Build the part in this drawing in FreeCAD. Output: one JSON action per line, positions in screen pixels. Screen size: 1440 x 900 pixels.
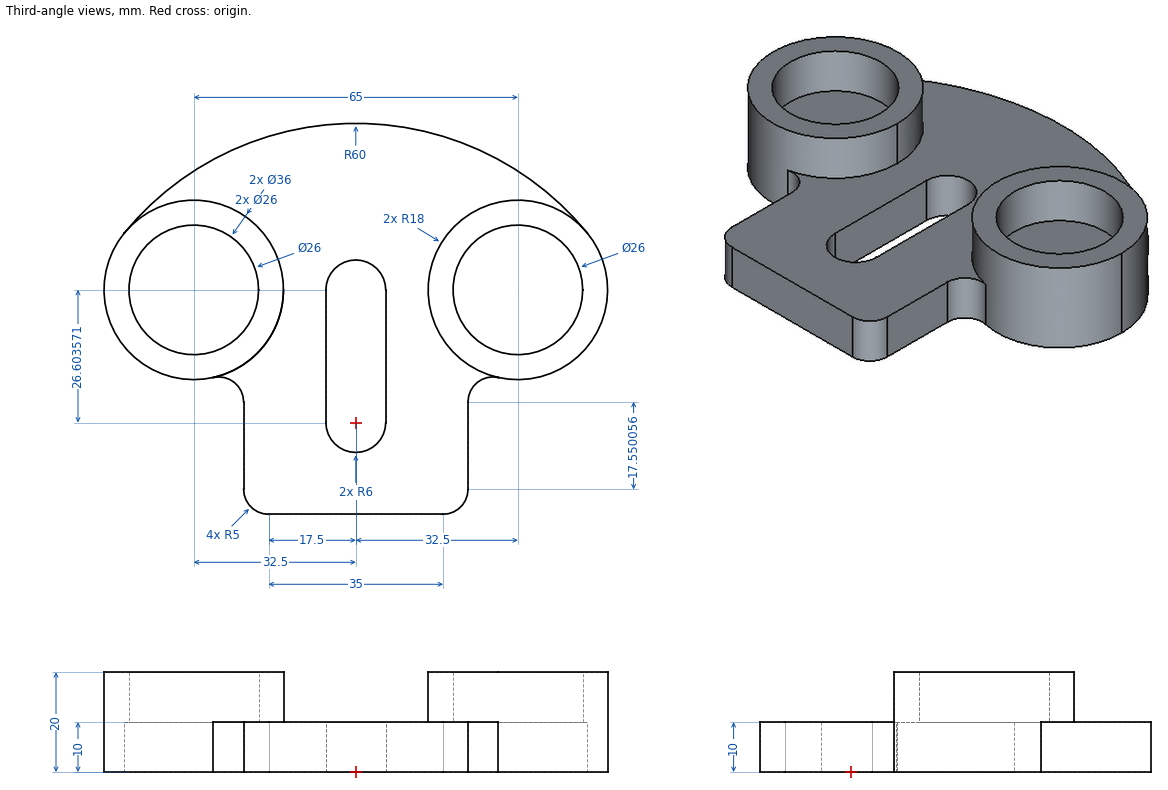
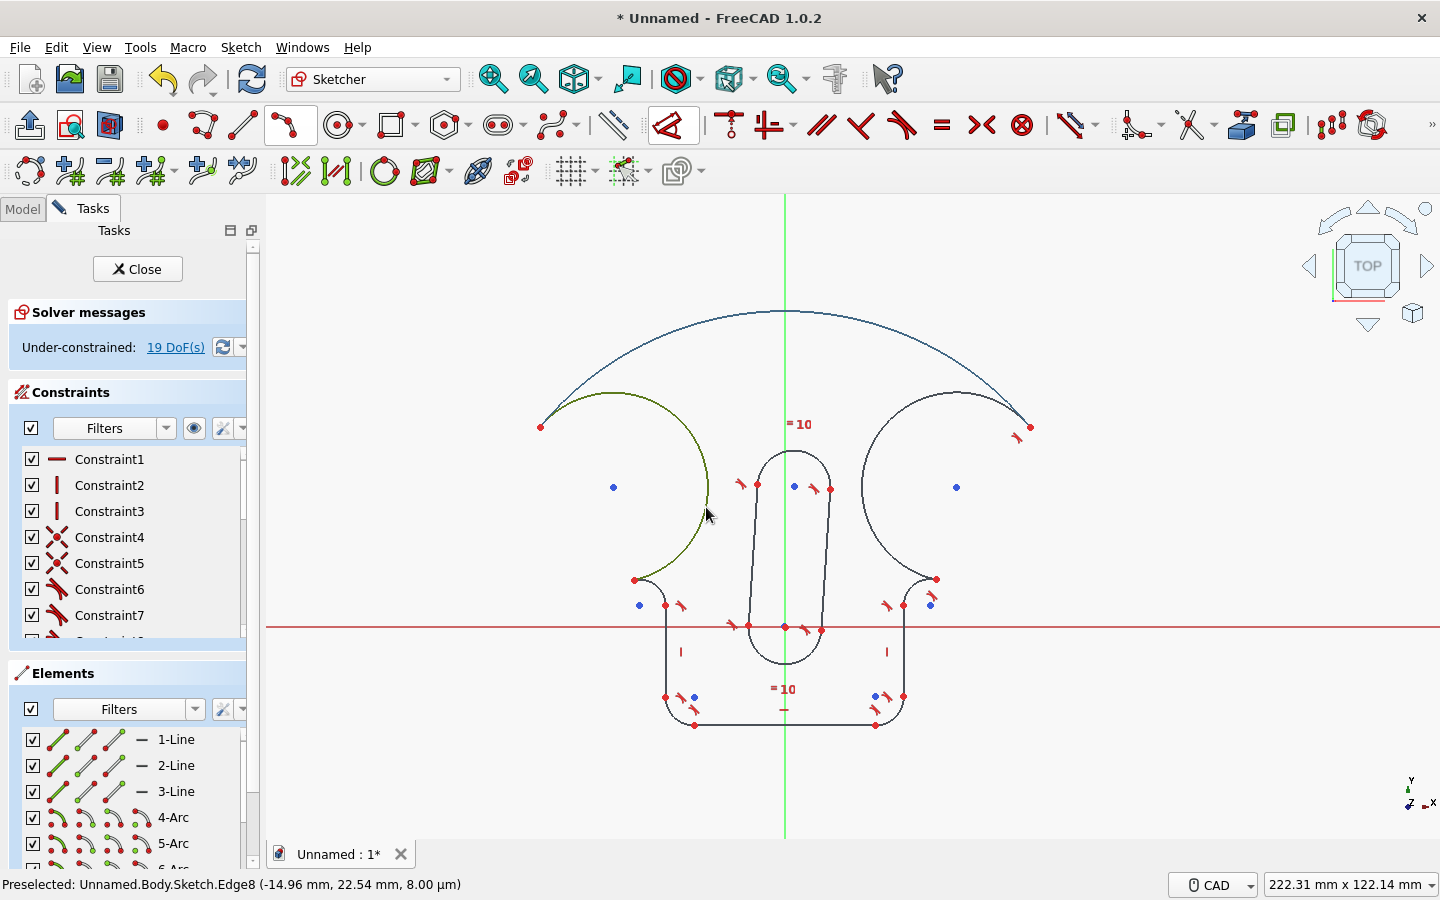
{"action": "left_click", "coordinate": [902, 126]}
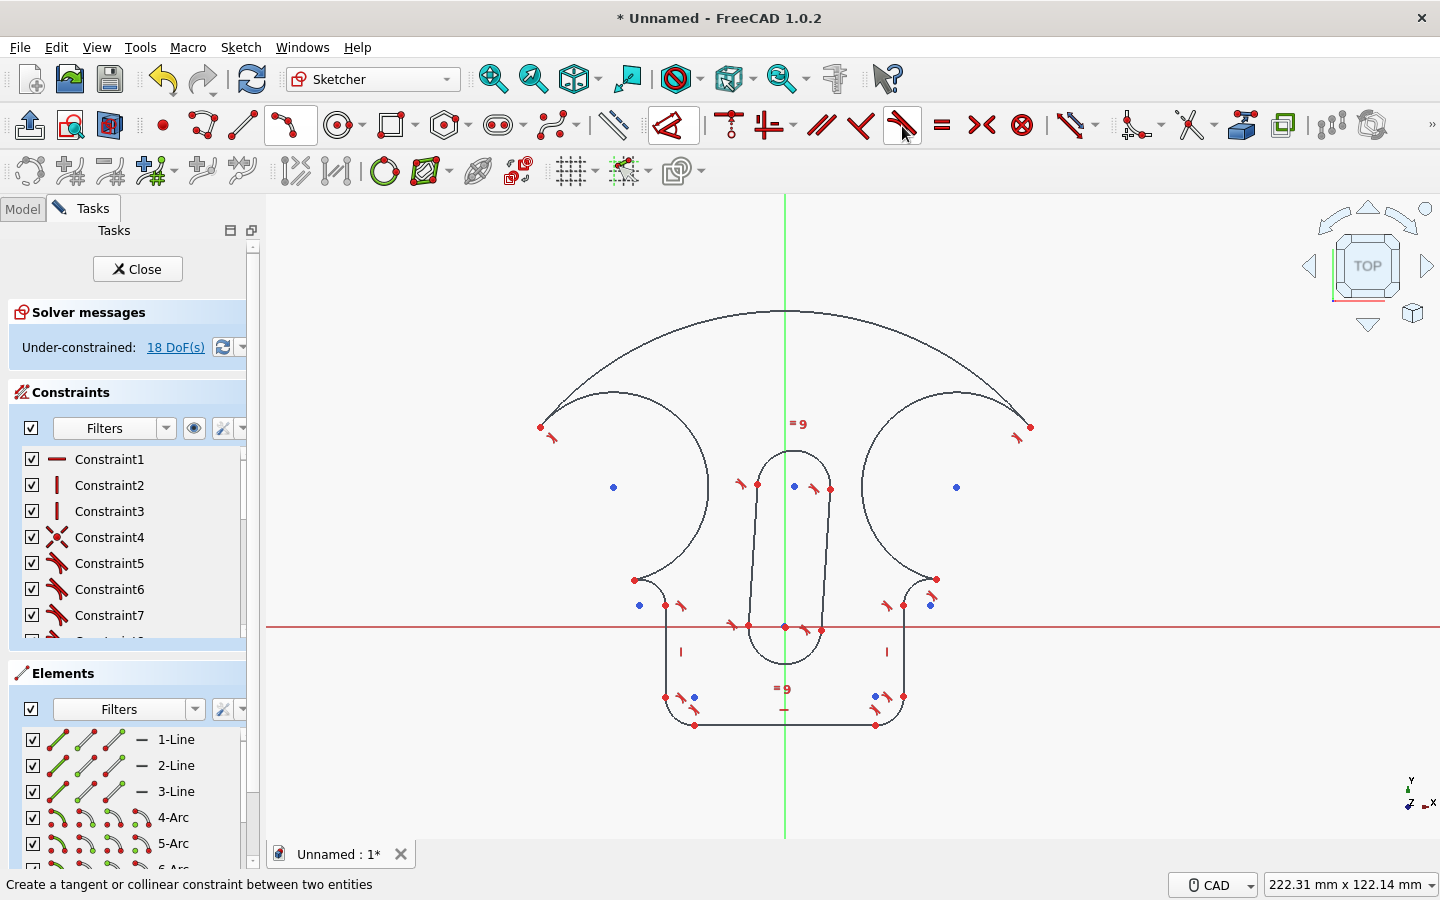
{"action": "left_click", "coordinate": [706, 507]}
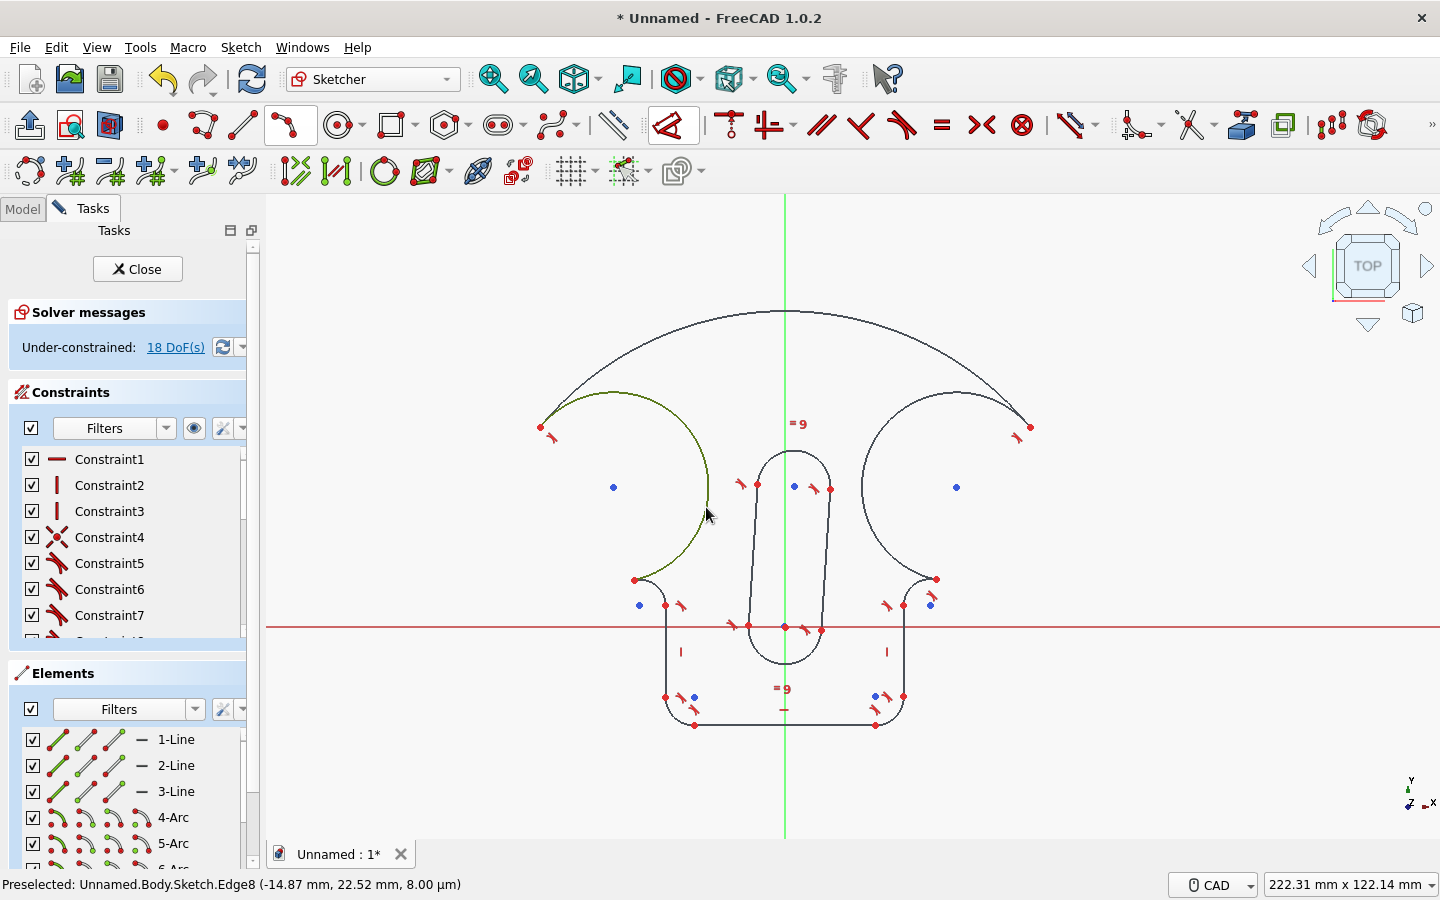
{"action": "left_click", "coordinate": [662, 592]}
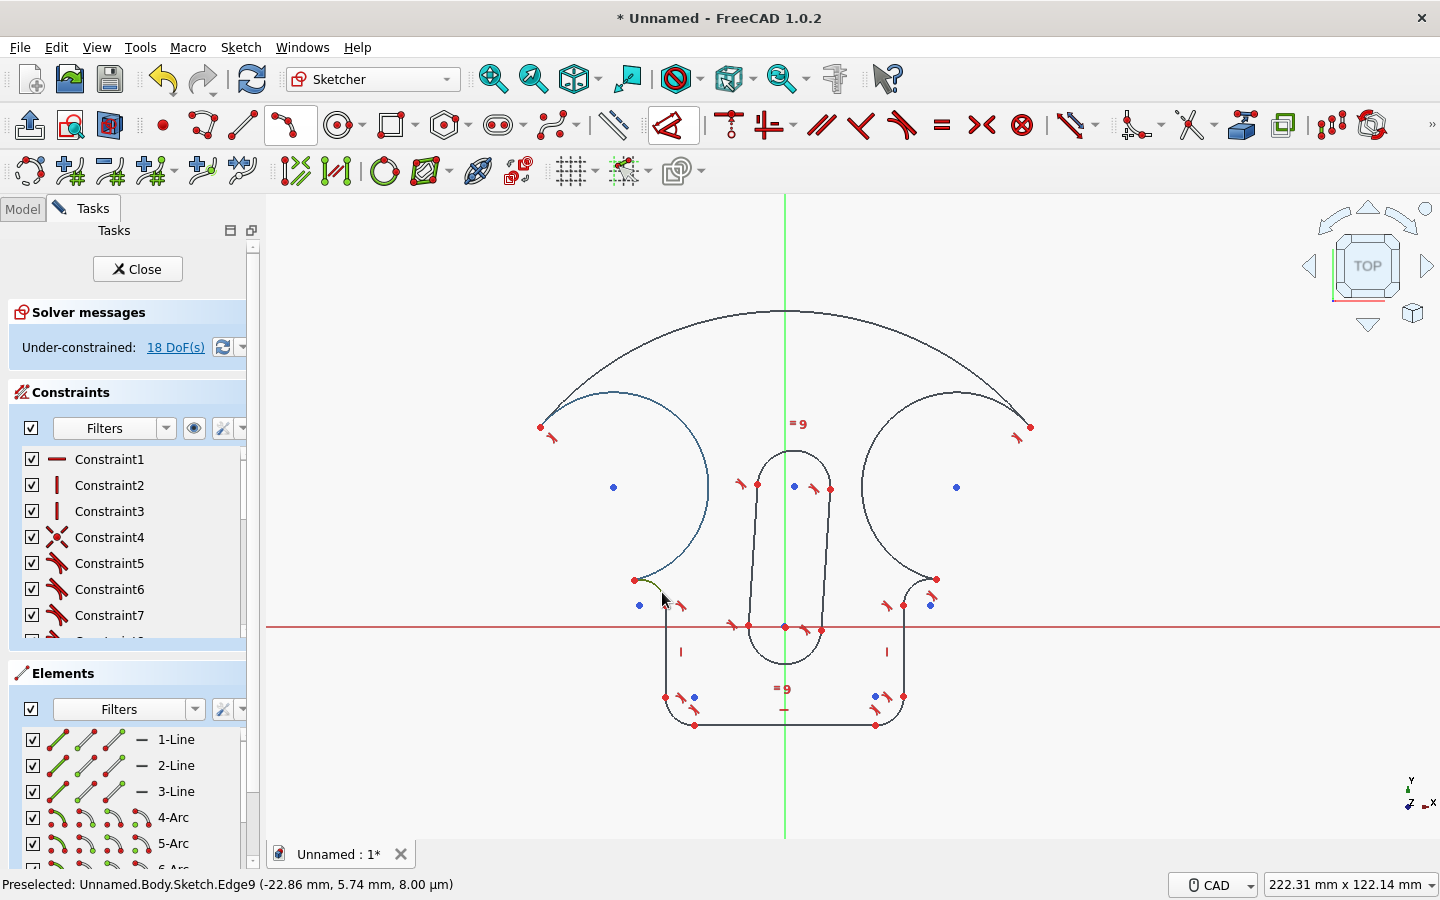
{"action": "left_click", "coordinate": [902, 126]}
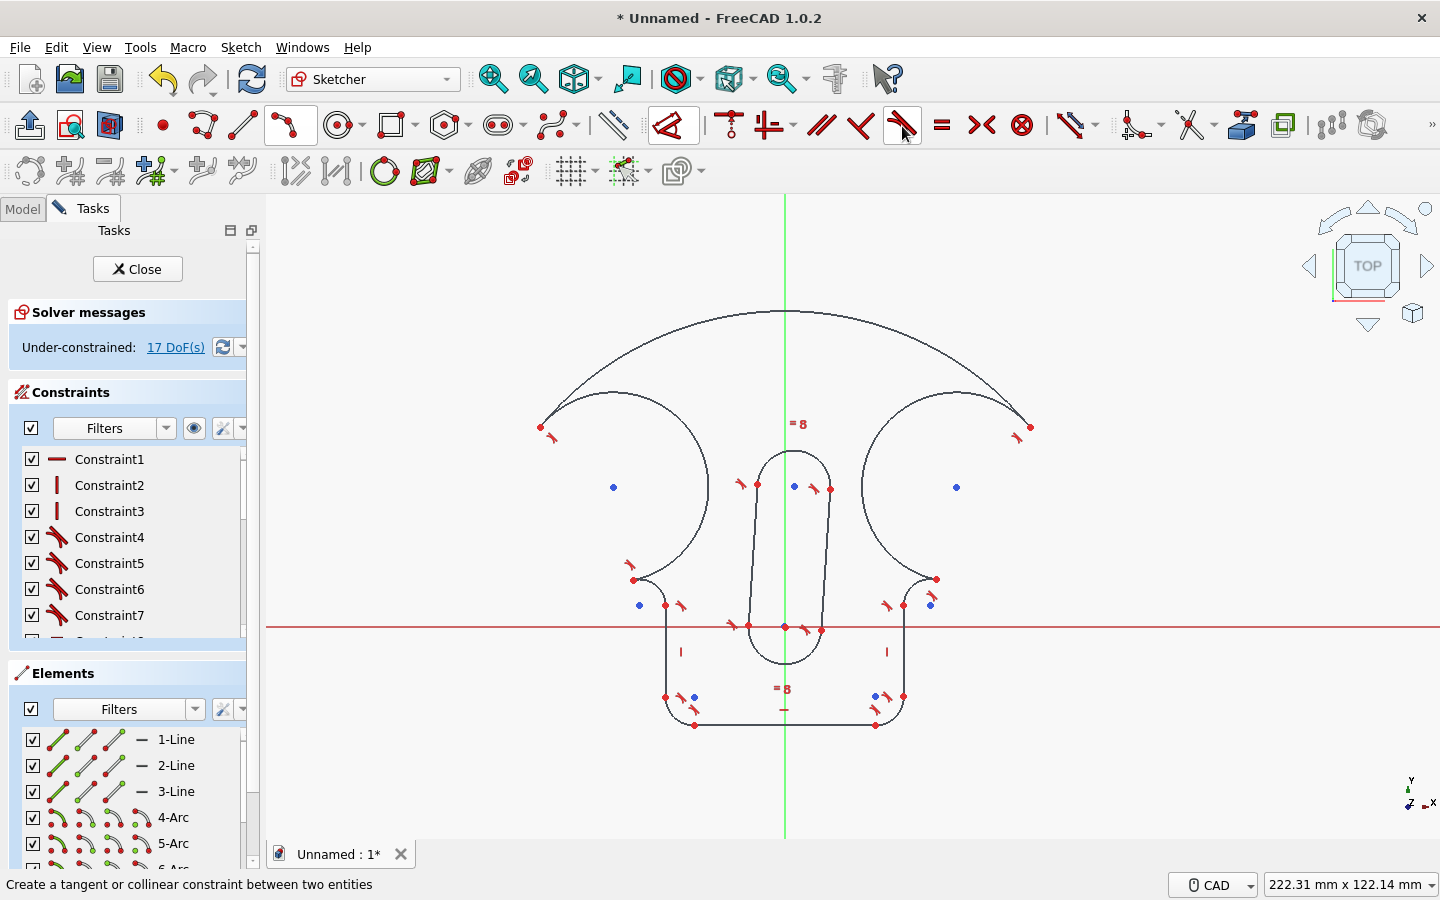
{"action": "left_click", "coordinate": [751, 583]}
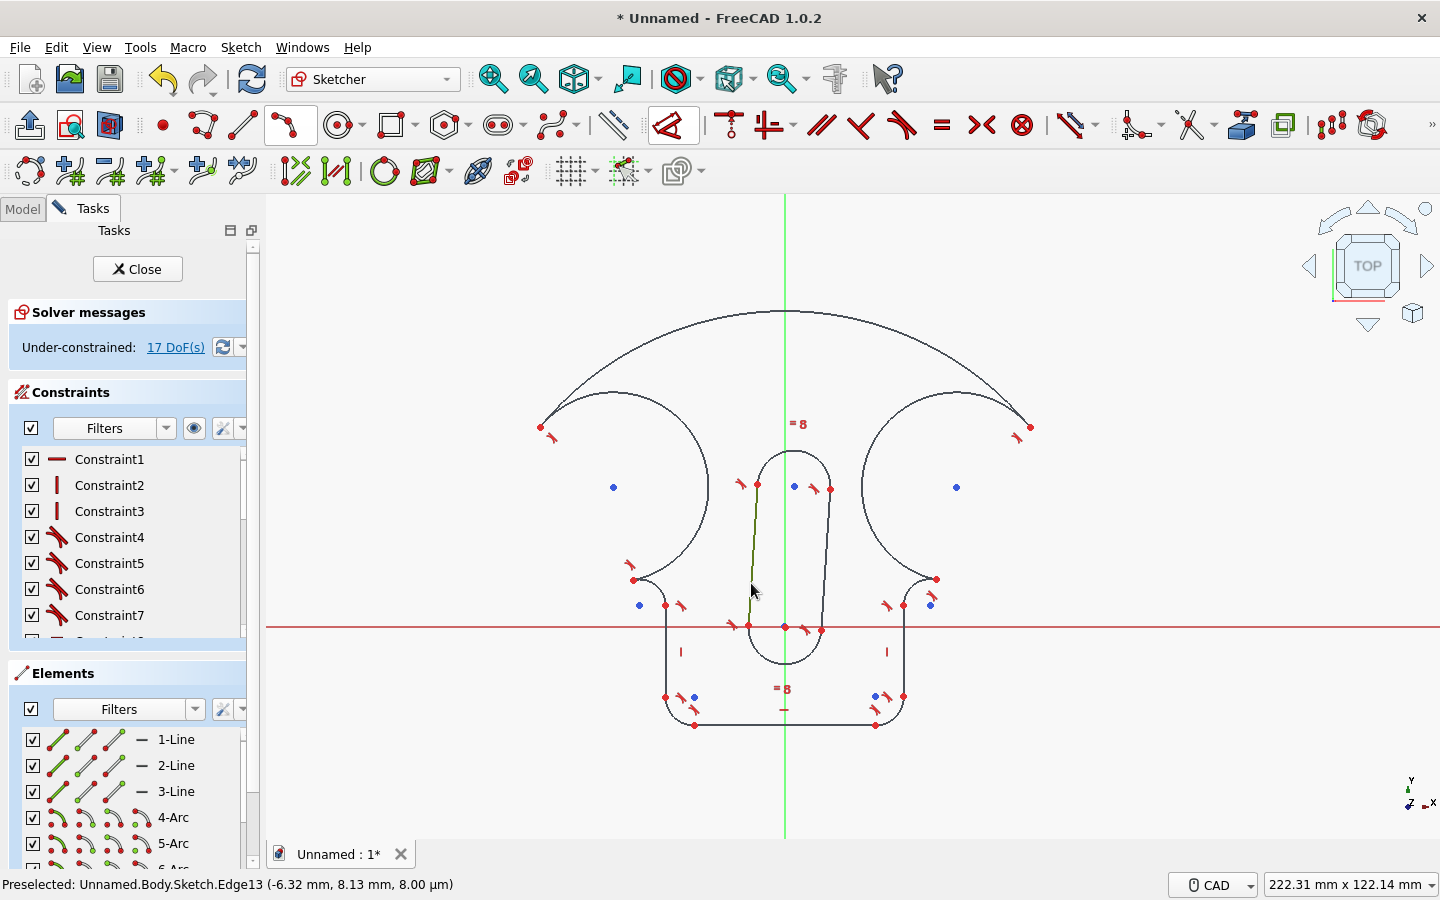
{"action": "left_click", "coordinate": [796, 126]}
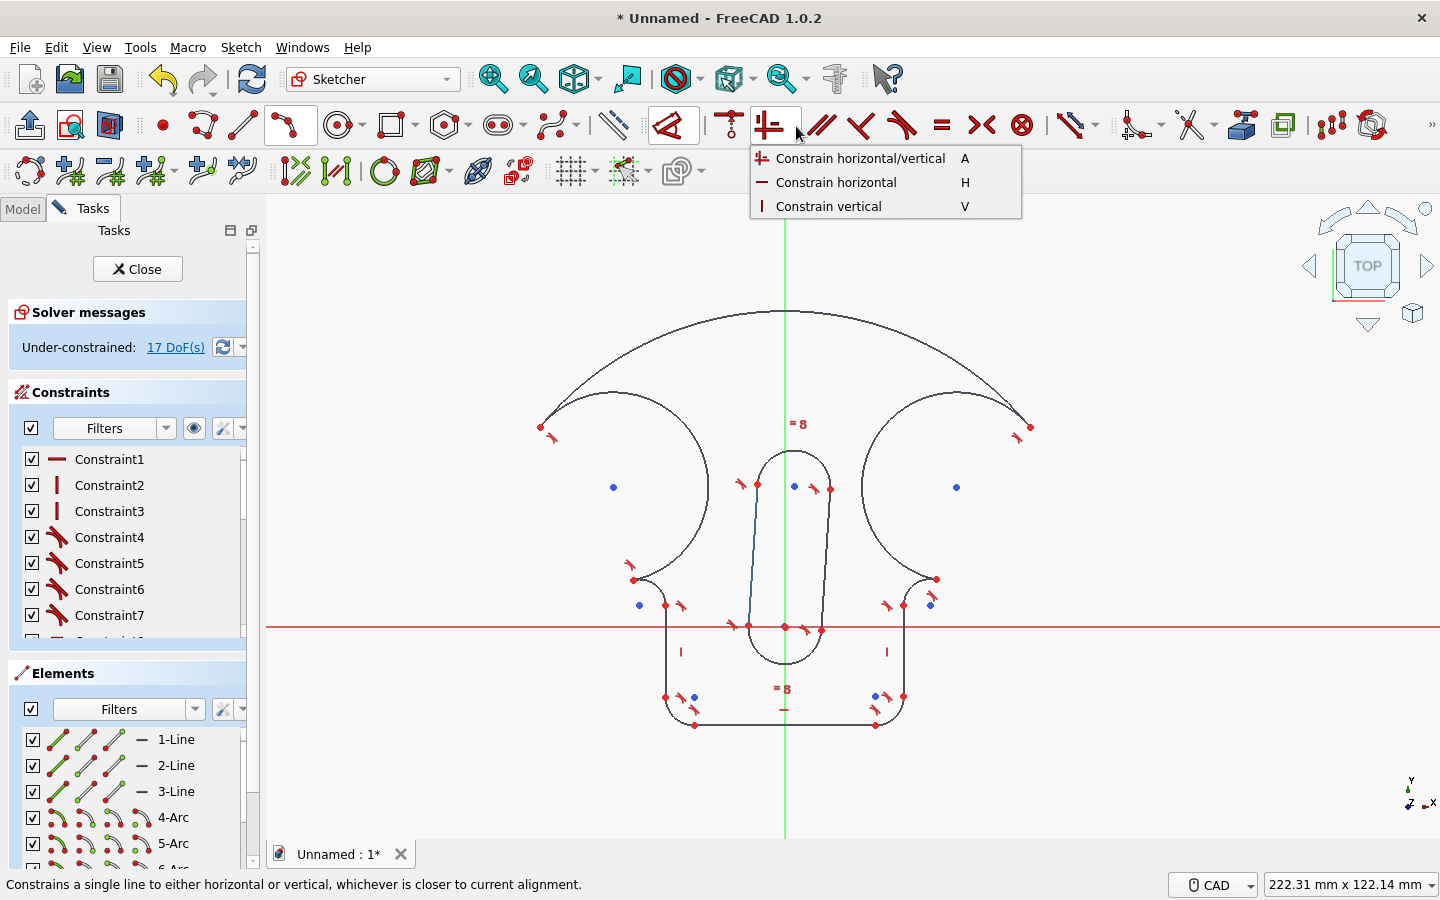
{"action": "left_click", "coordinate": [886, 206]}